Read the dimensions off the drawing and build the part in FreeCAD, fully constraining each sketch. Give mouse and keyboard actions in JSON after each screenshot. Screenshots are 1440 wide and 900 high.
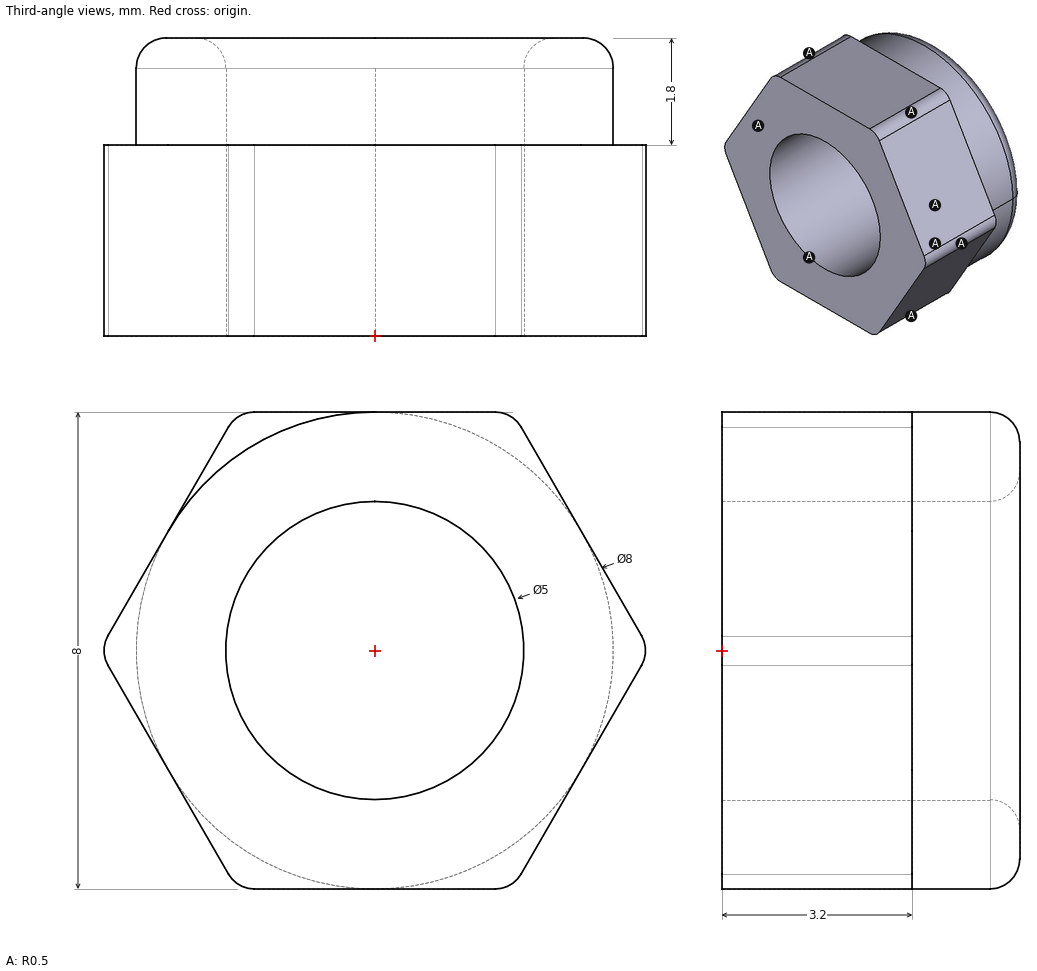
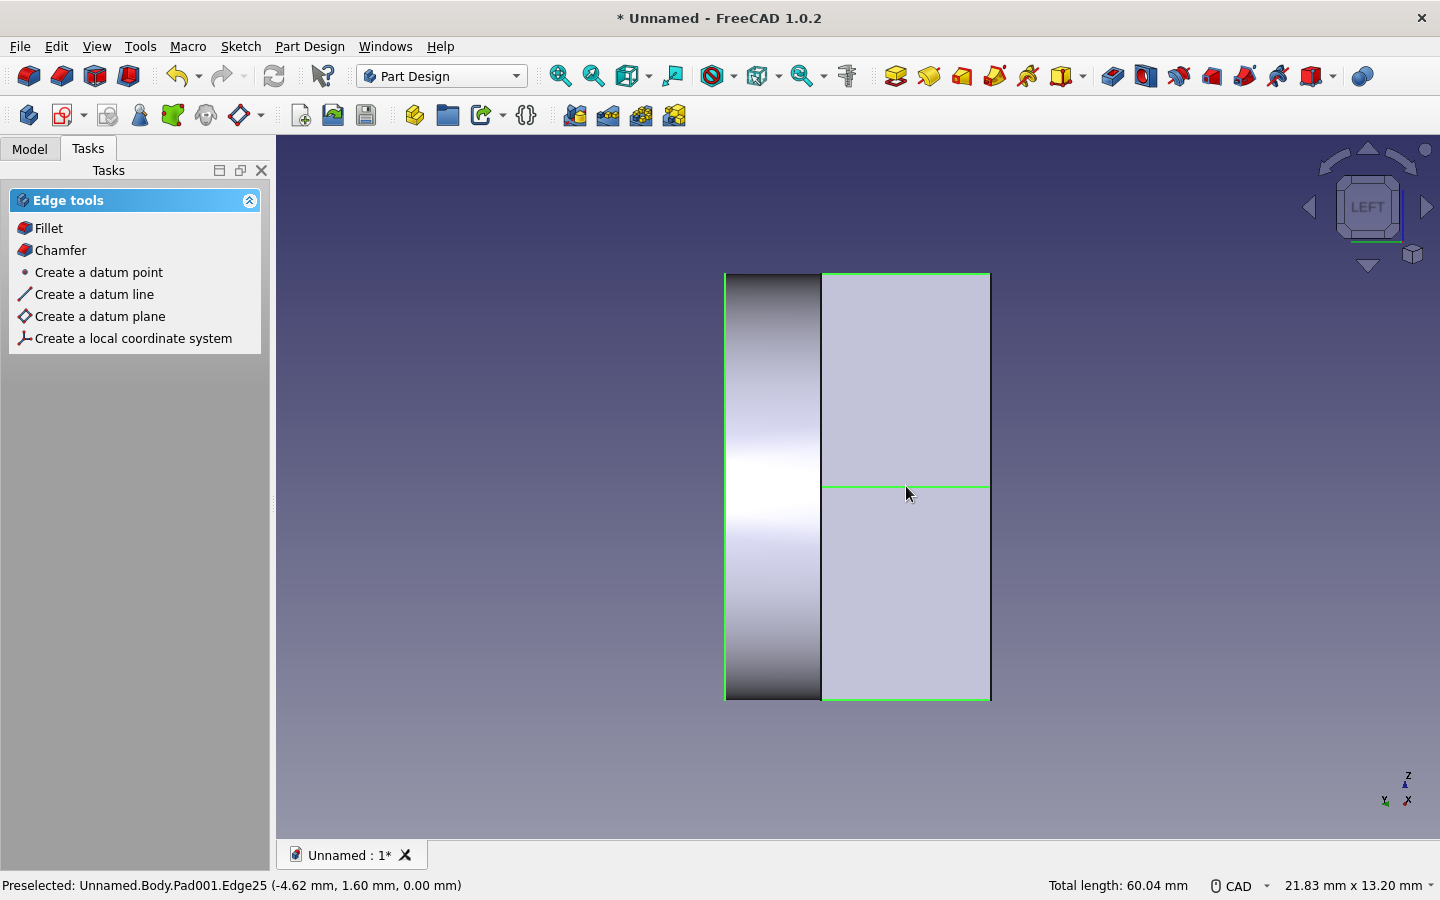
{"action": "left_click", "coordinate": [29, 76]}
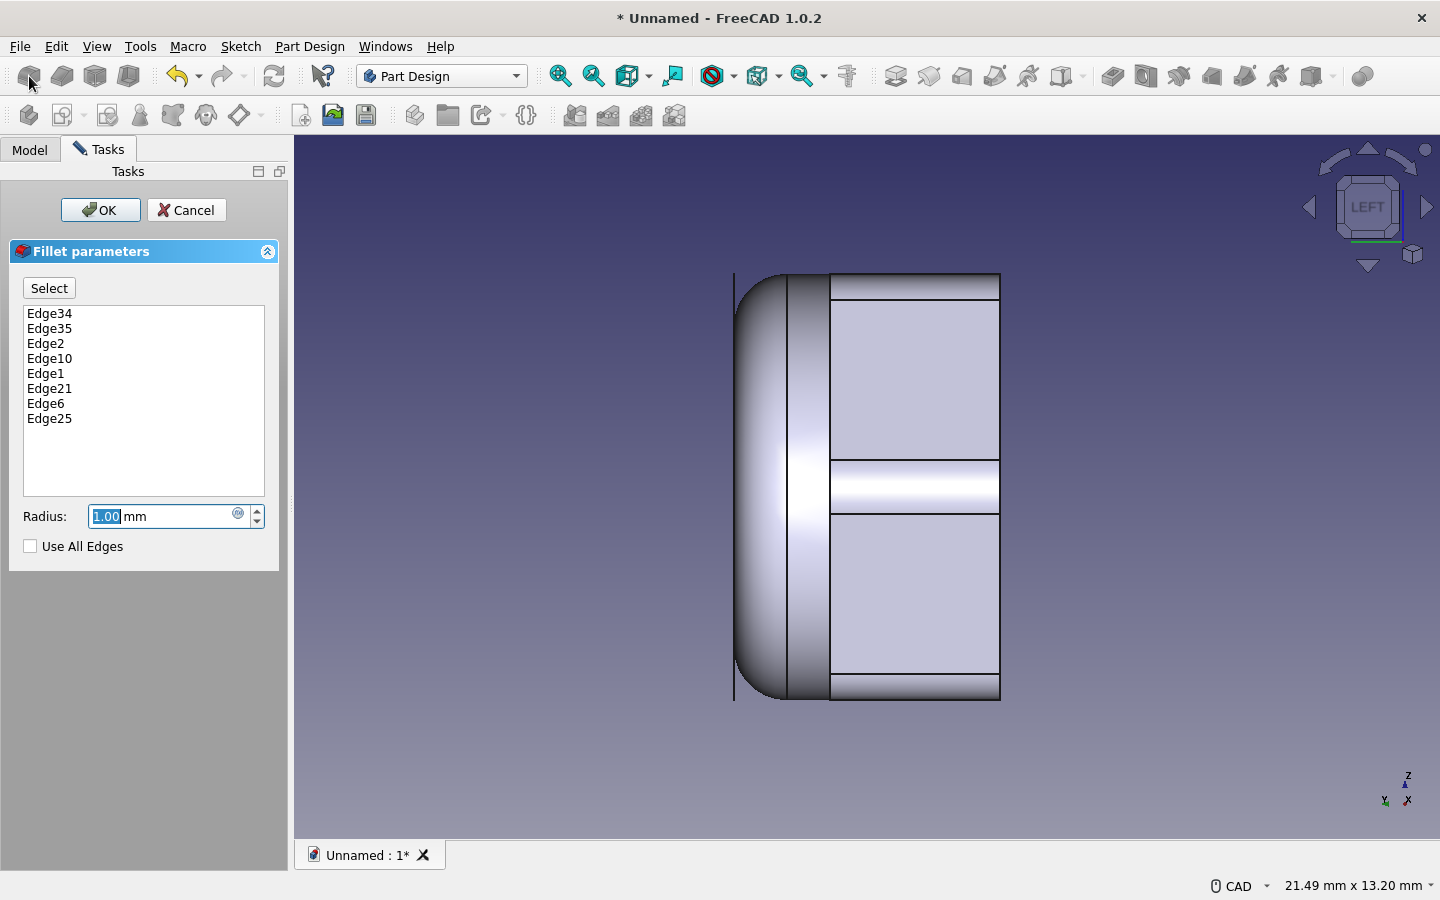
{"action": "type", "text": "0.5"}
{"action": "key", "text": "Tab"}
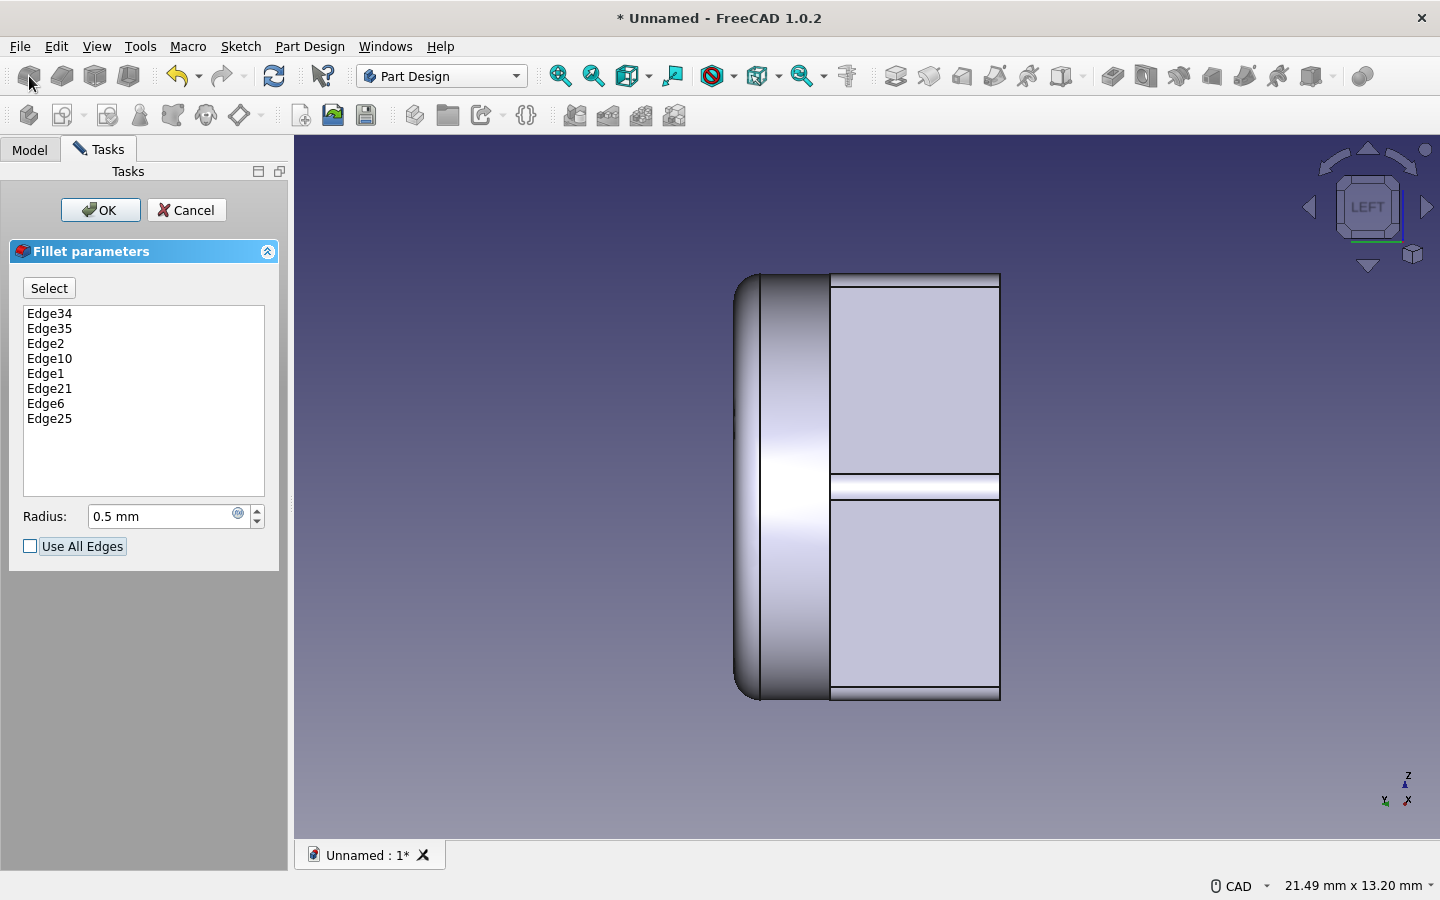
{"action": "left_click", "coordinate": [101, 210]}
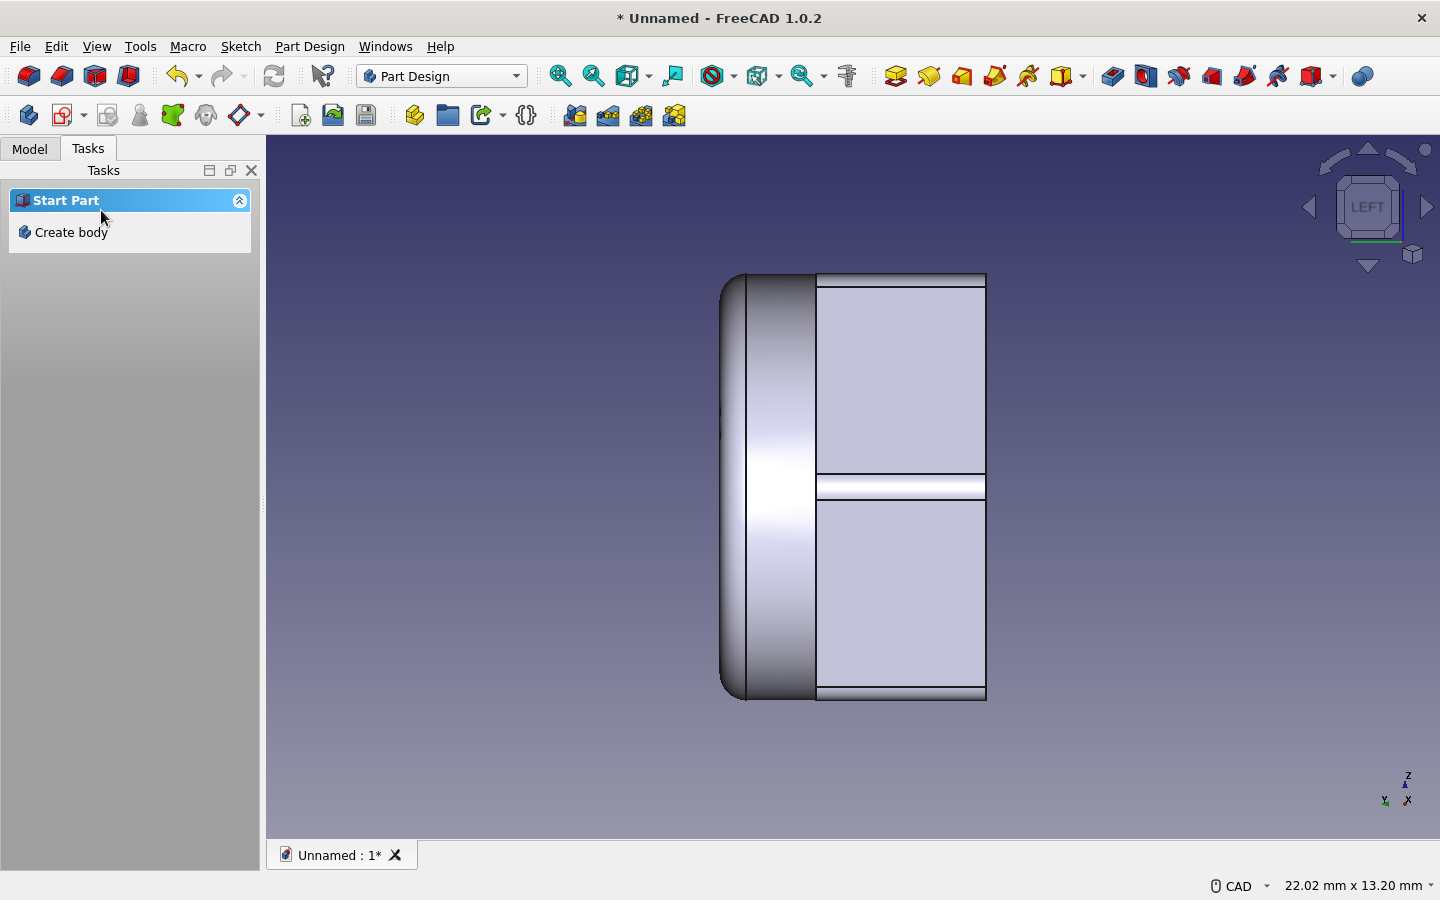
{"action": "key", "text": "0"}